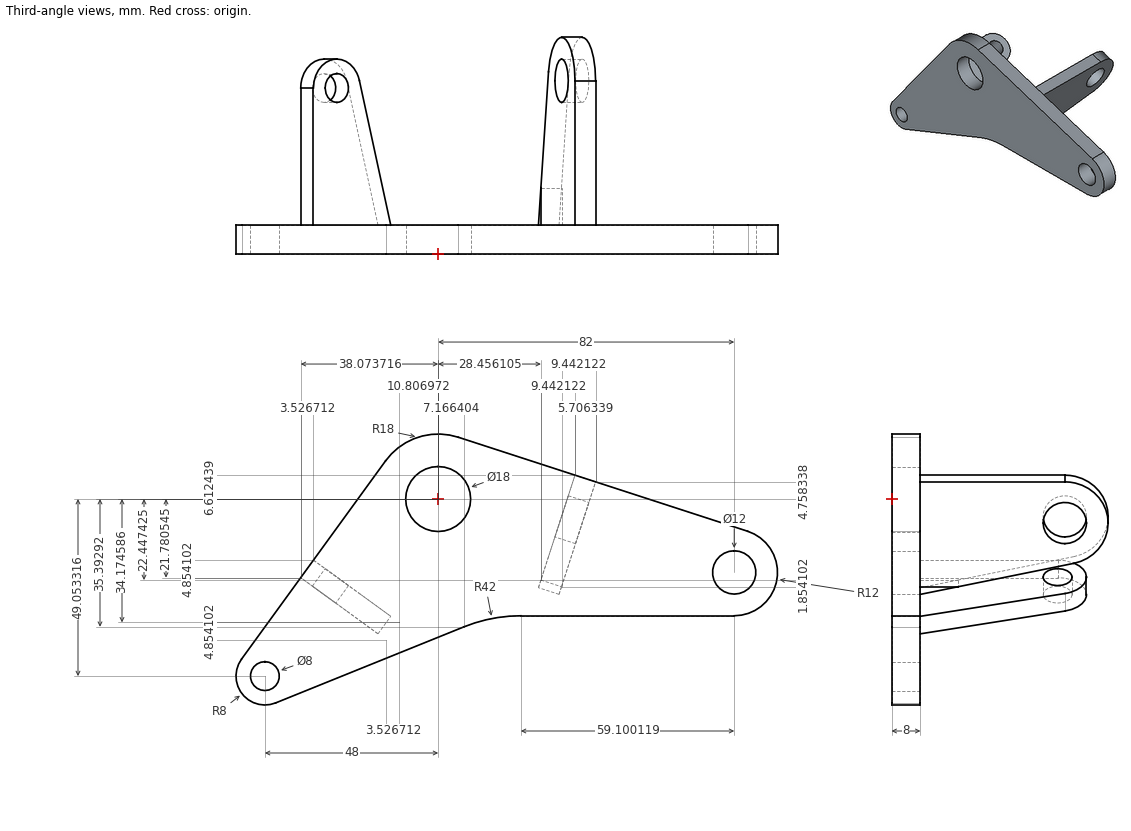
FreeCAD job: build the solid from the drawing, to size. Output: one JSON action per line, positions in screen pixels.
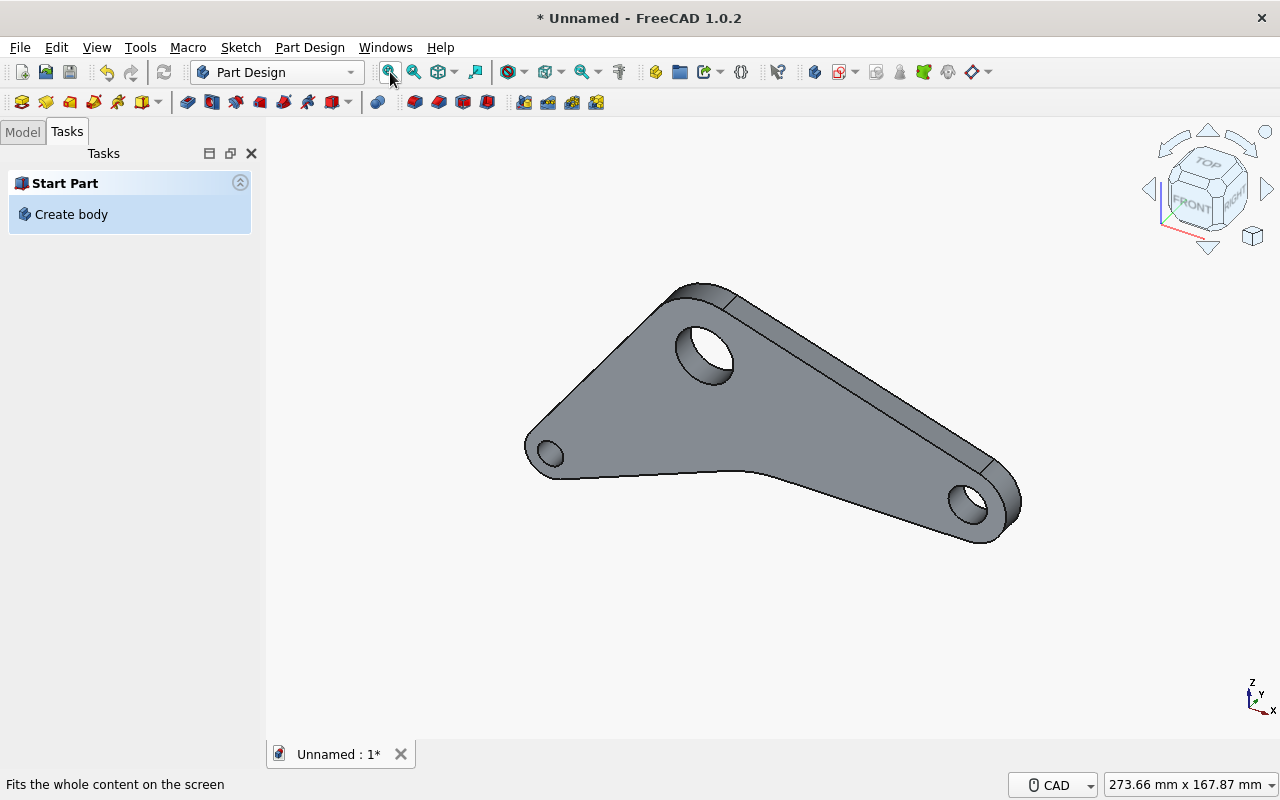
{"action": "key", "text": "4"}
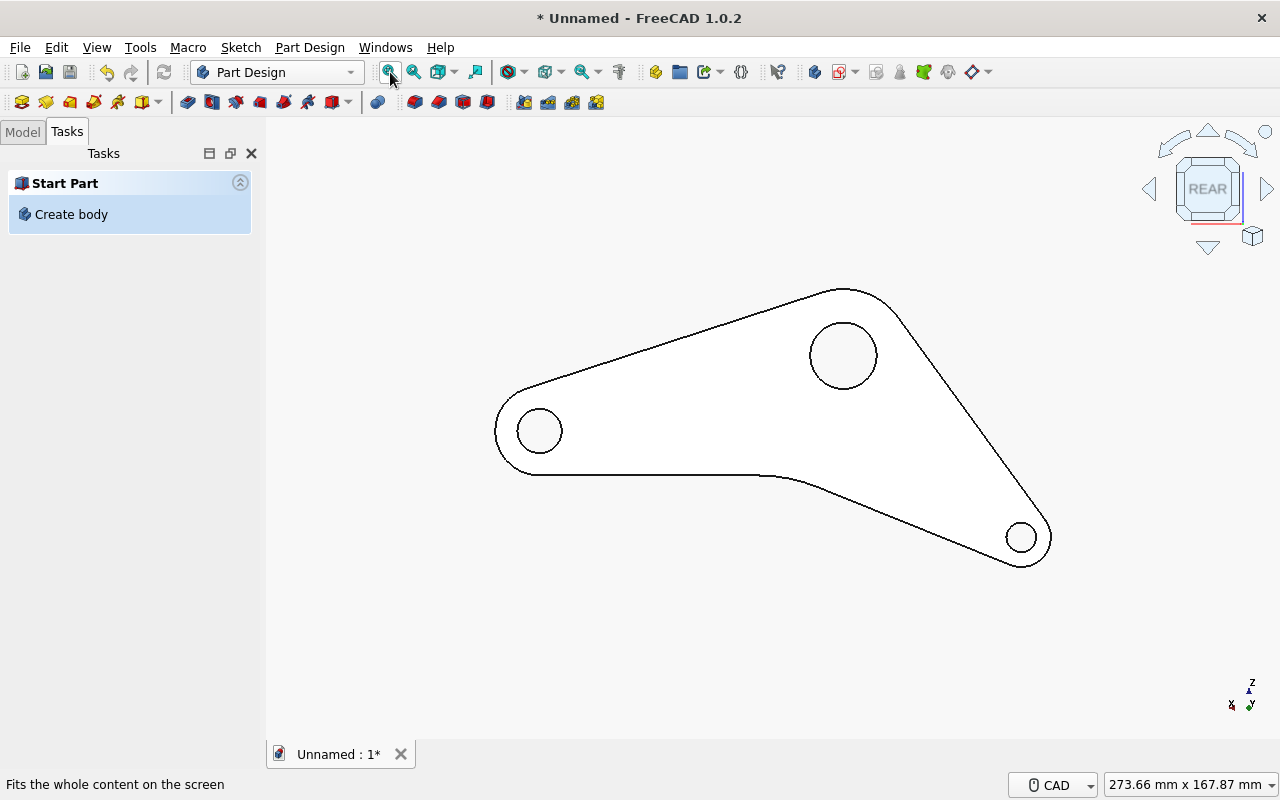
{"action": "left_click", "coordinate": [932, 467]}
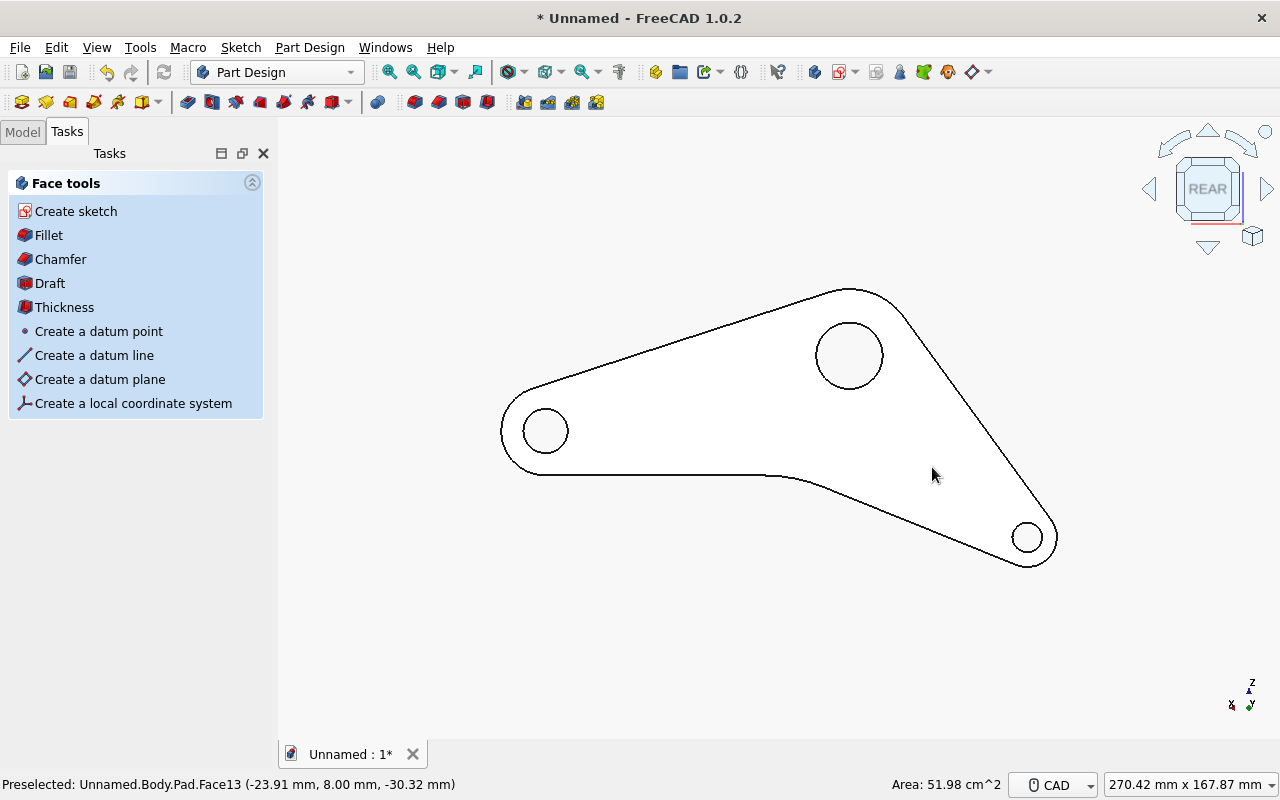
{"action": "left_click", "coordinate": [840, 72]}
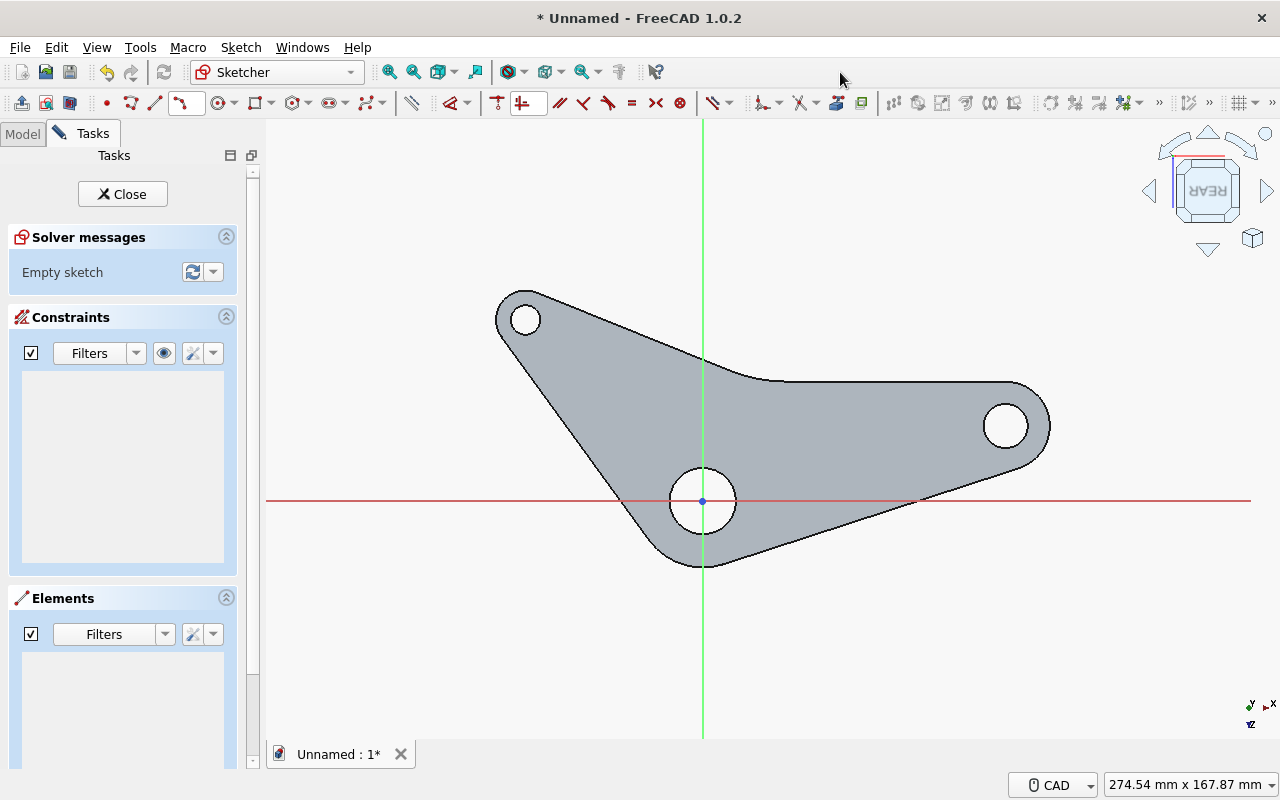
{"action": "scroll", "coordinate": [723, 456], "scroll_direction": "up", "scroll_amount": 3}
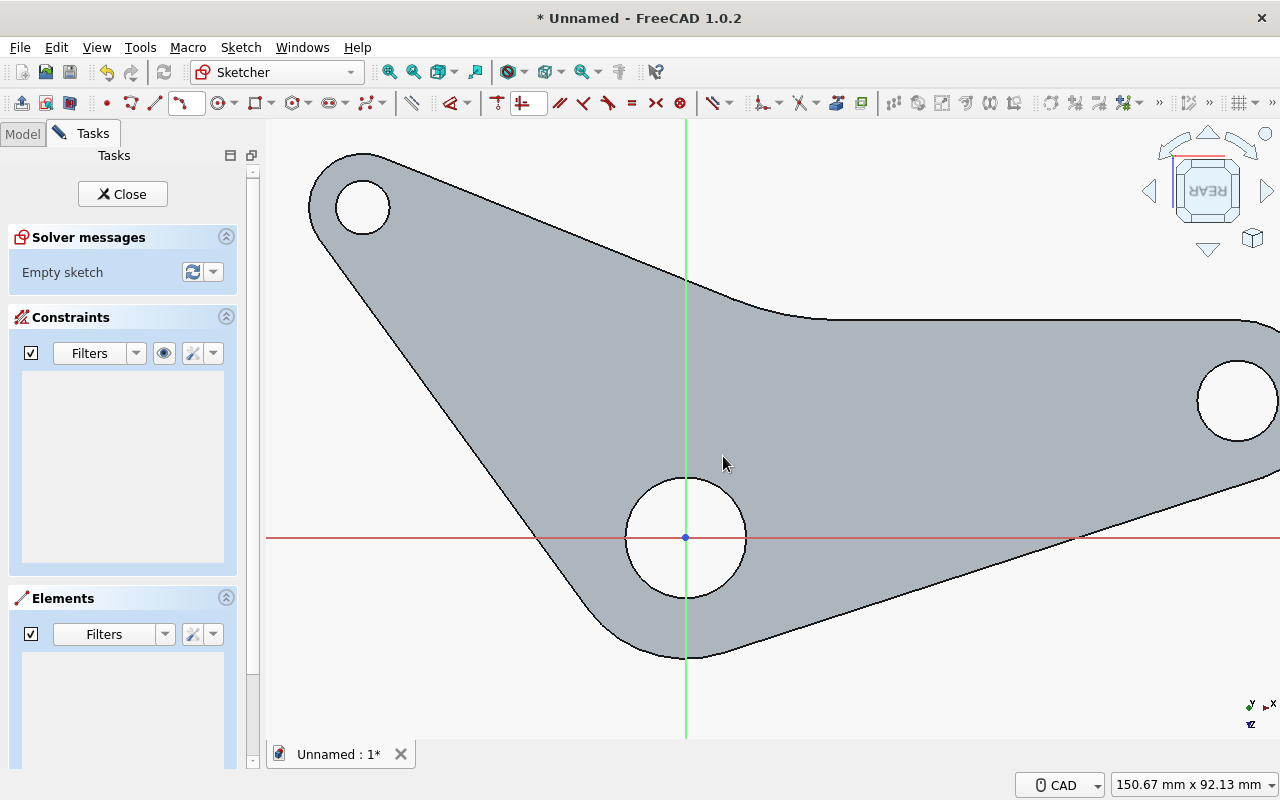
{"action": "left_click", "coordinate": [132, 104]}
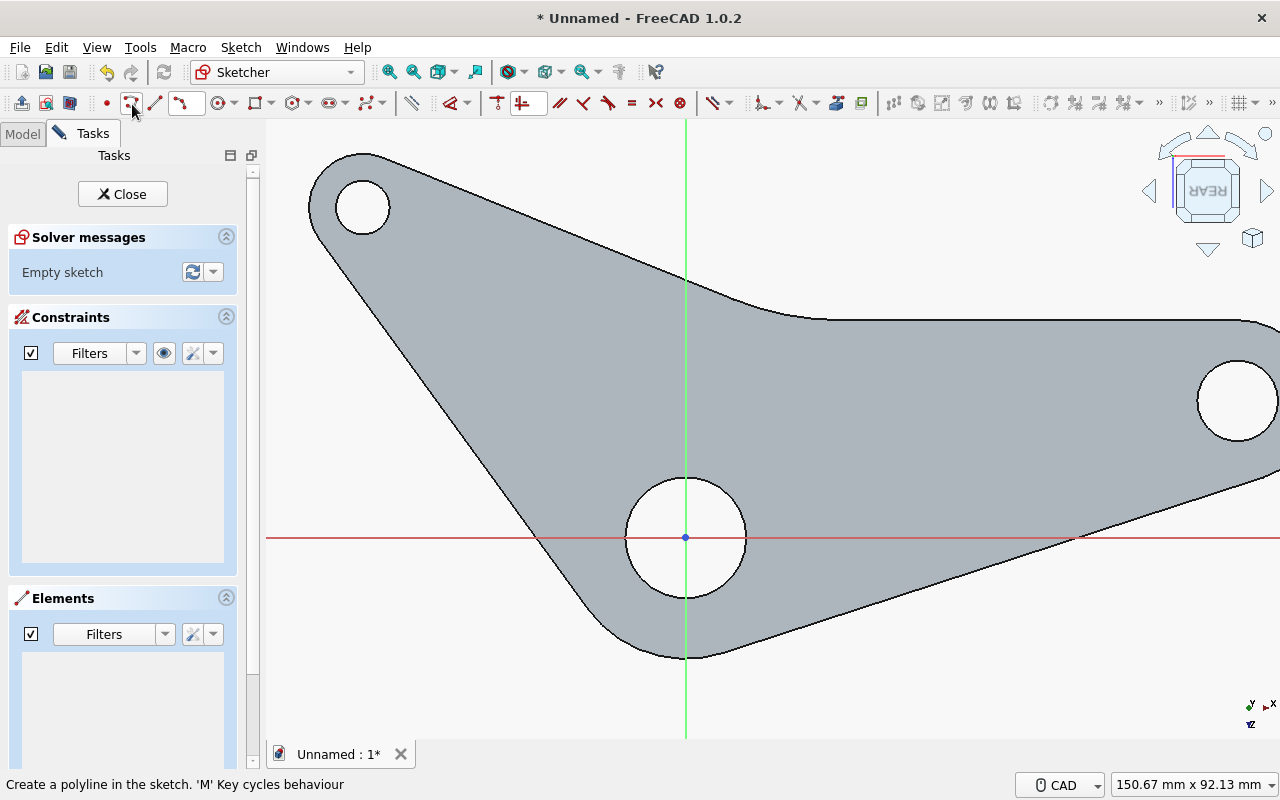
{"action": "left_click", "coordinate": [613, 308]}
{"action": "left_click", "coordinate": [589, 275]}
{"action": "left_click", "coordinate": [430, 391]}
{"action": "left_click", "coordinate": [453, 424]}
{"action": "left_click", "coordinate": [613, 309]}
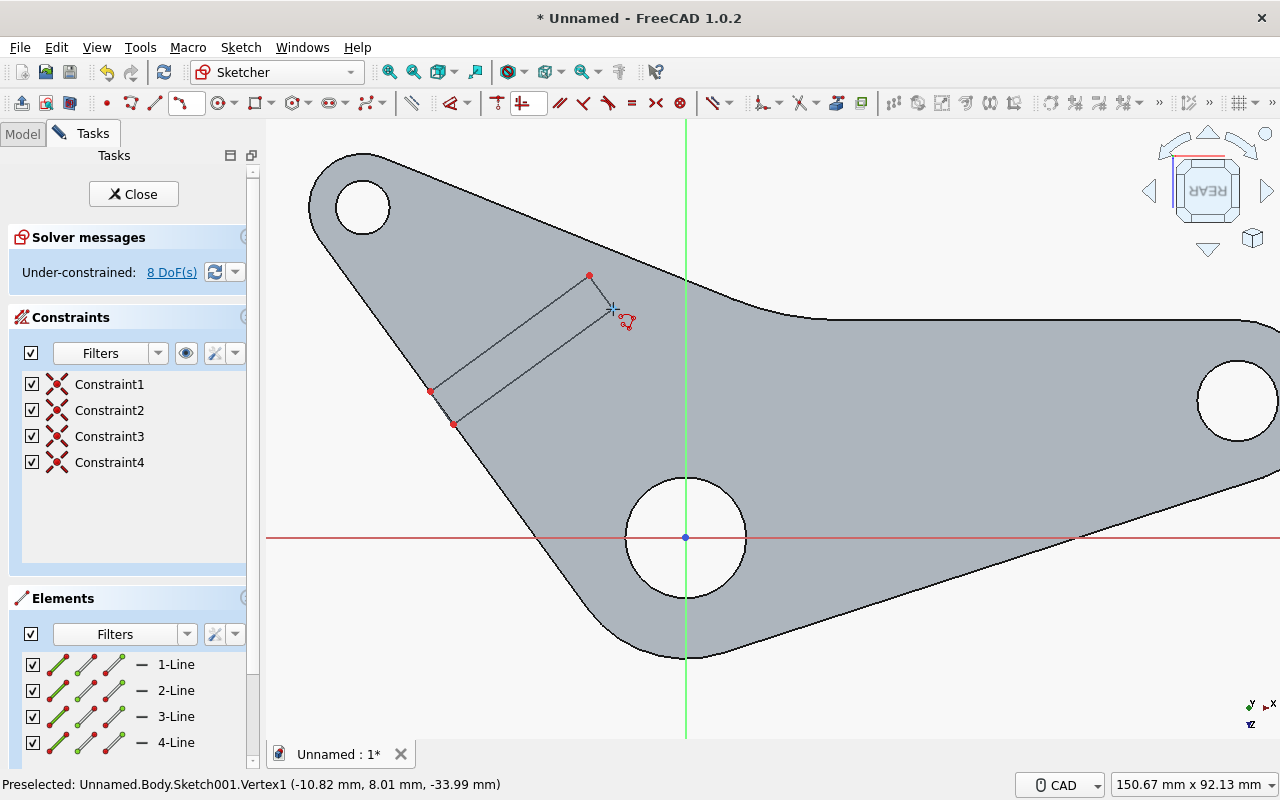
{"action": "left_click", "coordinate": [877, 387]}
{"action": "left_click", "coordinate": [941, 582]}
{"action": "left_click", "coordinate": [979, 570]}
{"action": "left_click", "coordinate": [916, 374]}
{"action": "left_click", "coordinate": [877, 388]}
{"action": "key", "text": "Escape"}
{"action": "key", "text": "Escape"}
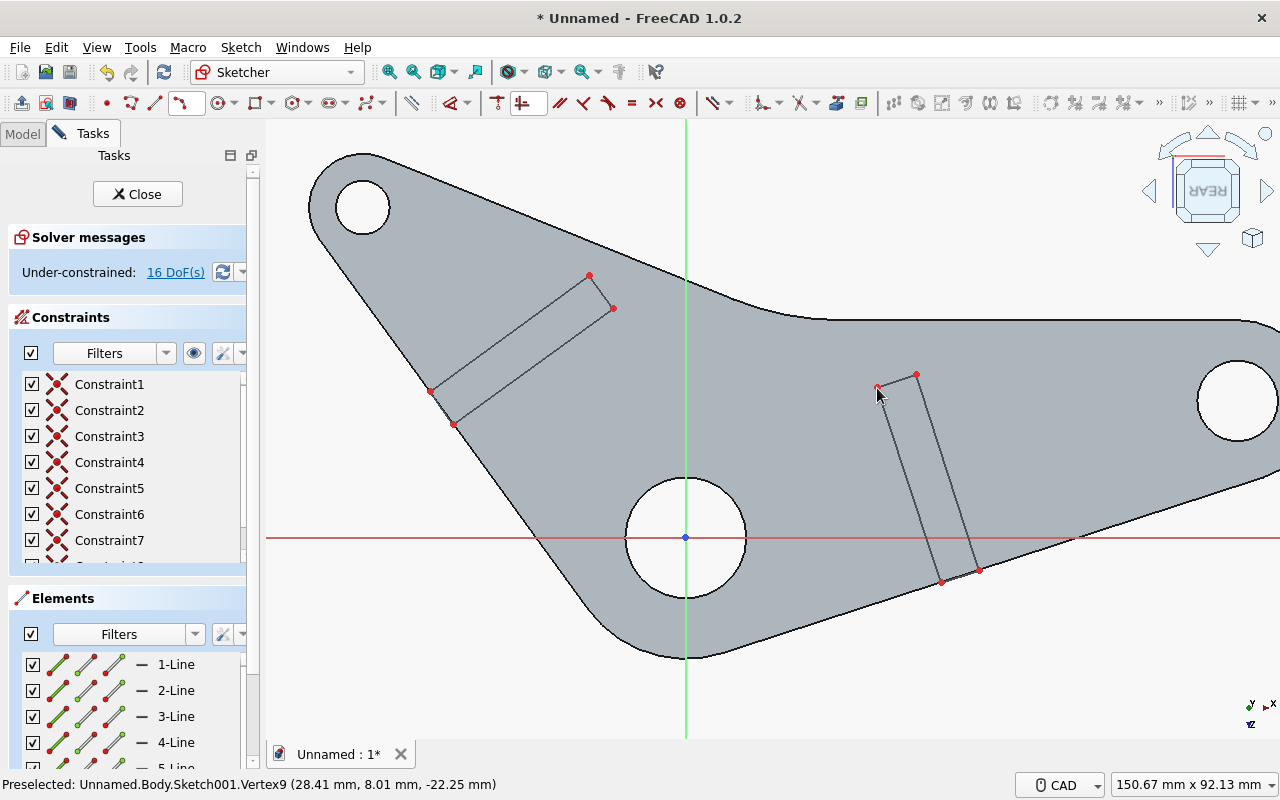
{"action": "left_click", "coordinate": [450, 104]}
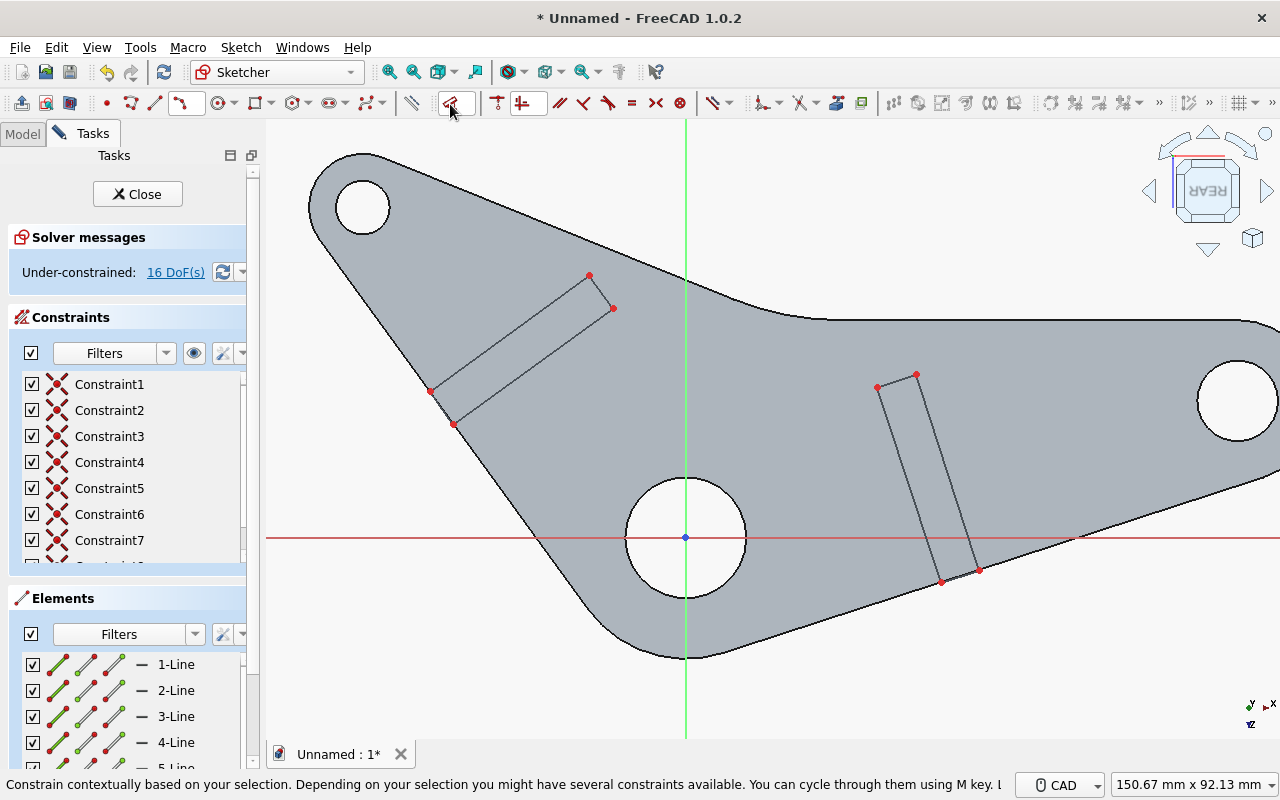
{"action": "left_click", "coordinate": [941, 583]}
{"action": "left_click", "coordinate": [652, 560]}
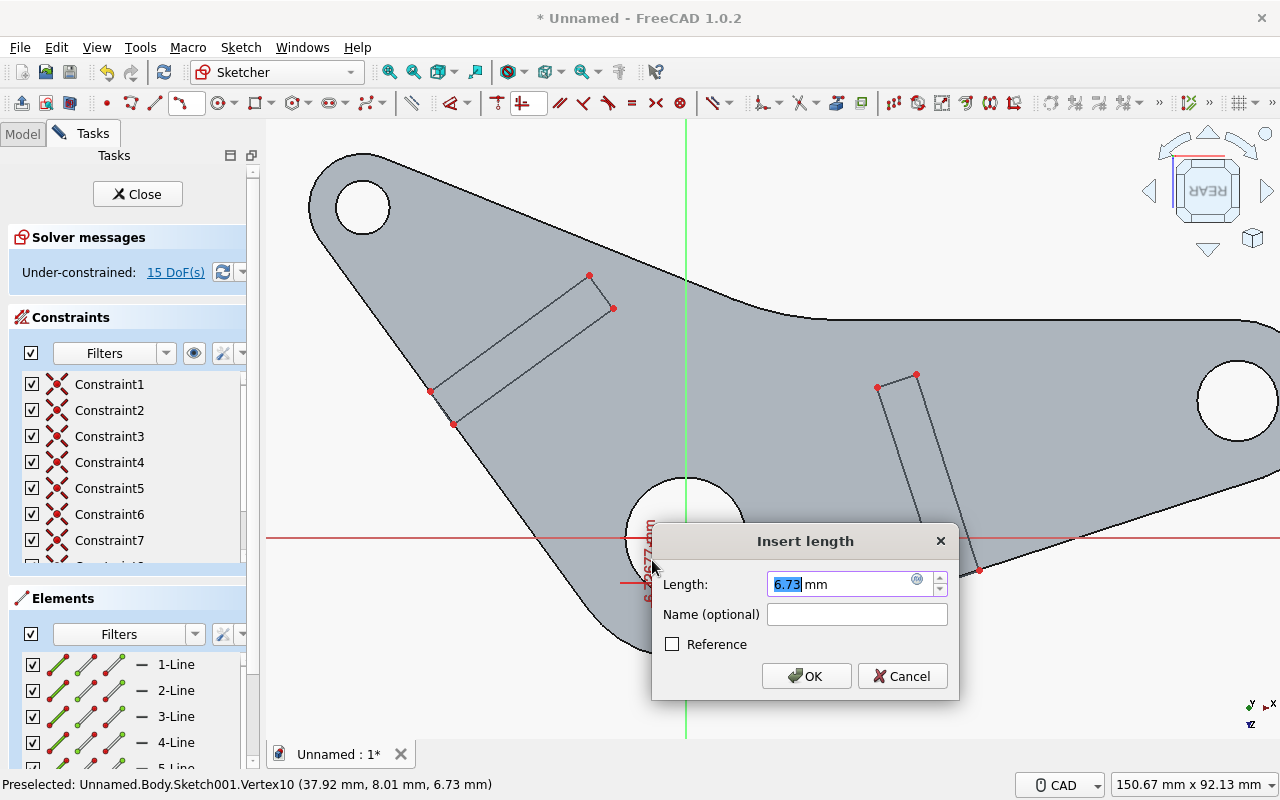
{"action": "type", "text": "6.612439"}
{"action": "key", "text": "Return"}